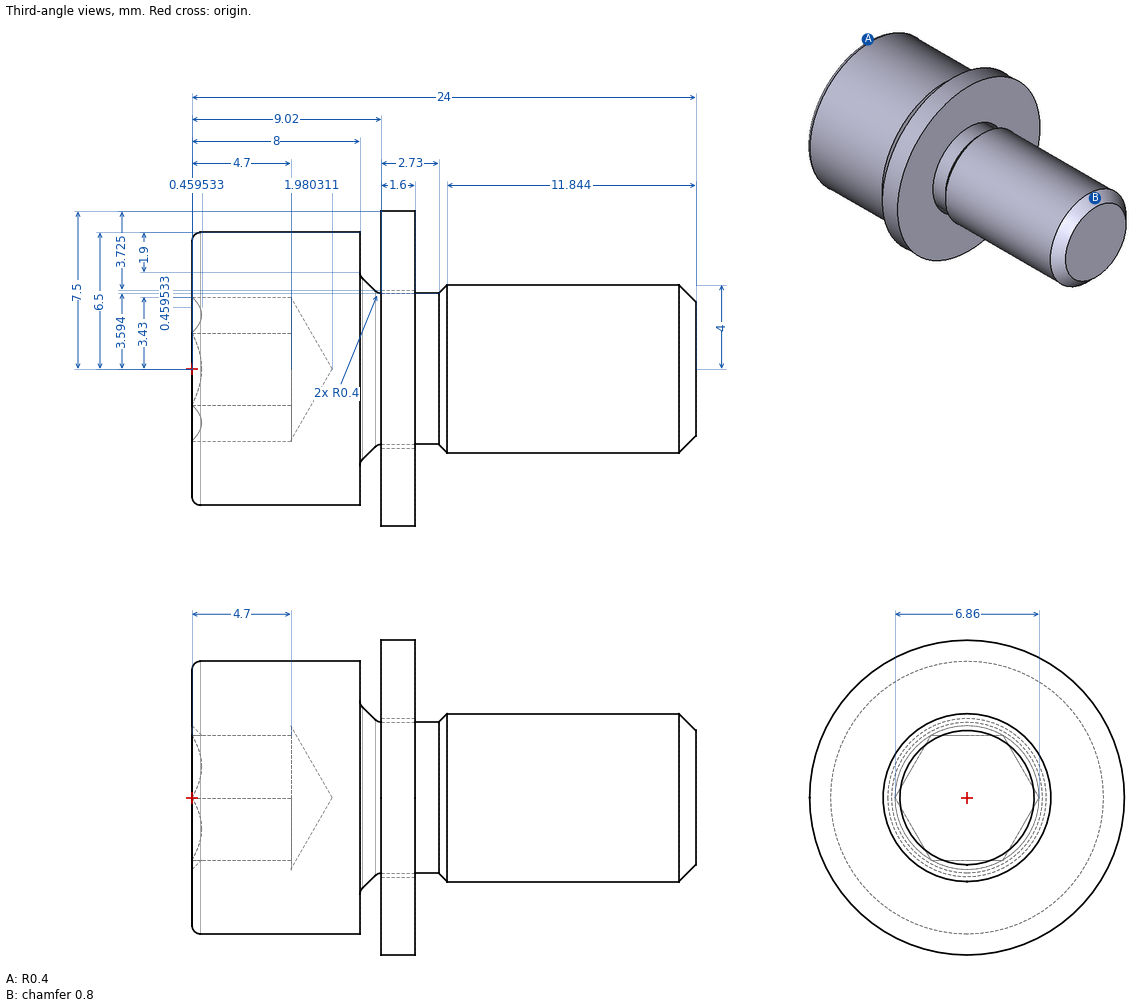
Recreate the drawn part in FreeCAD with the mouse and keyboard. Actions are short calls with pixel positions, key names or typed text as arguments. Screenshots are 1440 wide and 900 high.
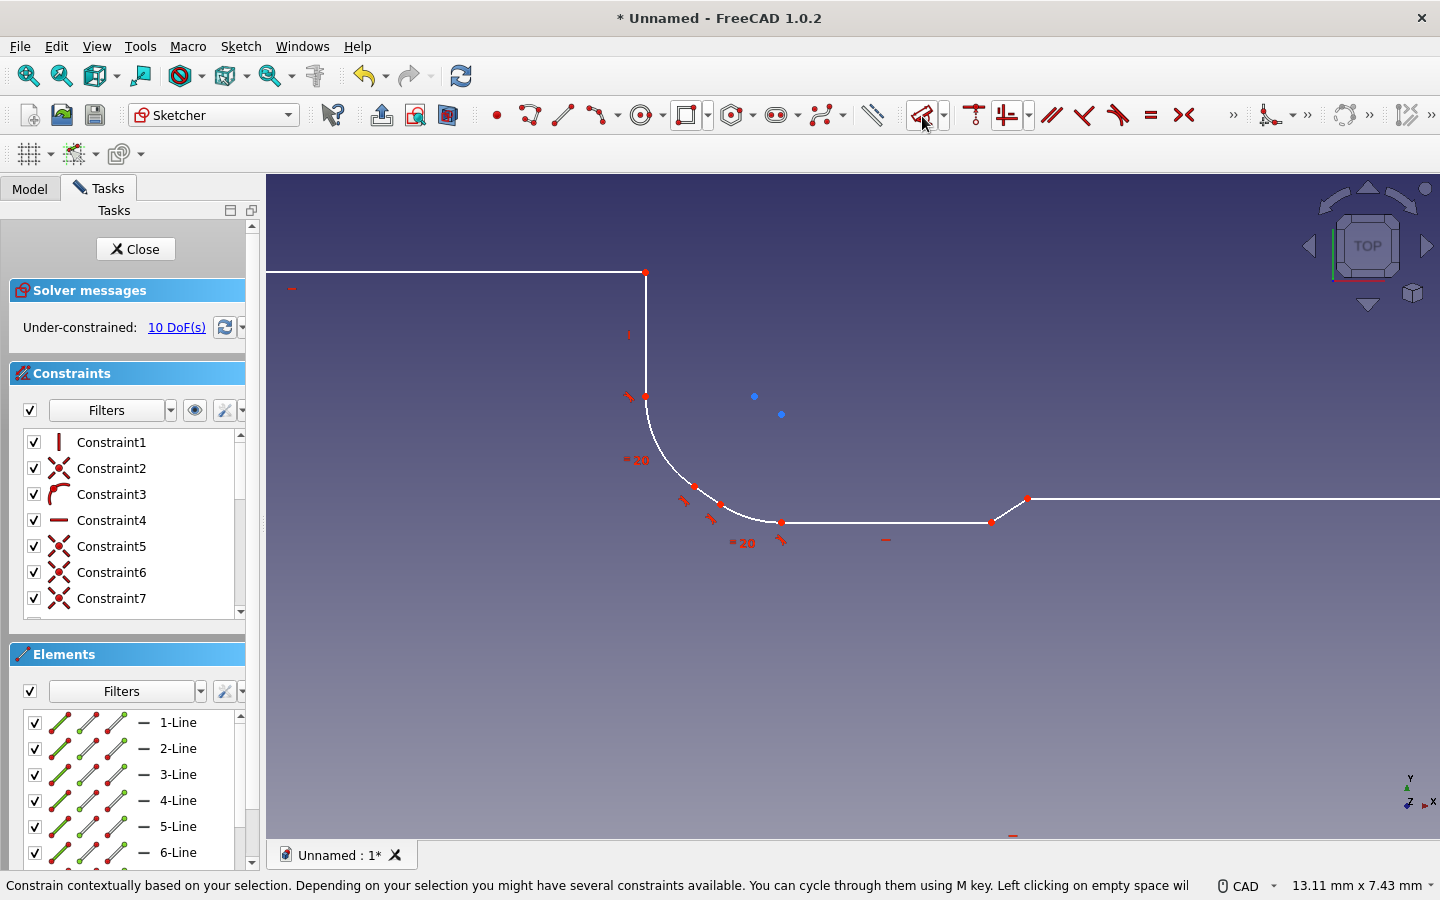
click(651, 428)
click(620, 437)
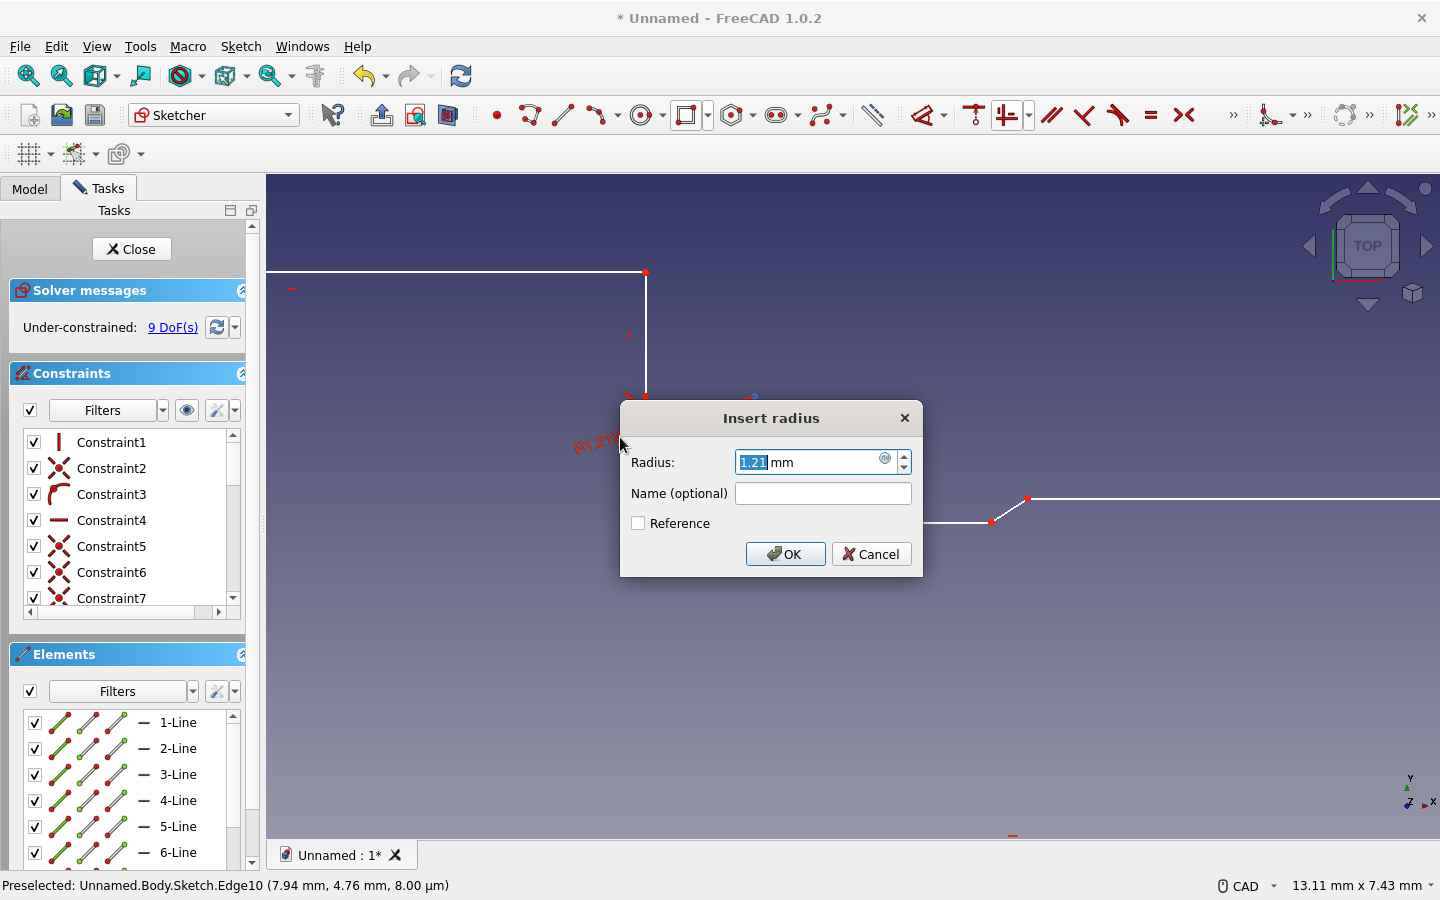
text(0.4)
key(Return)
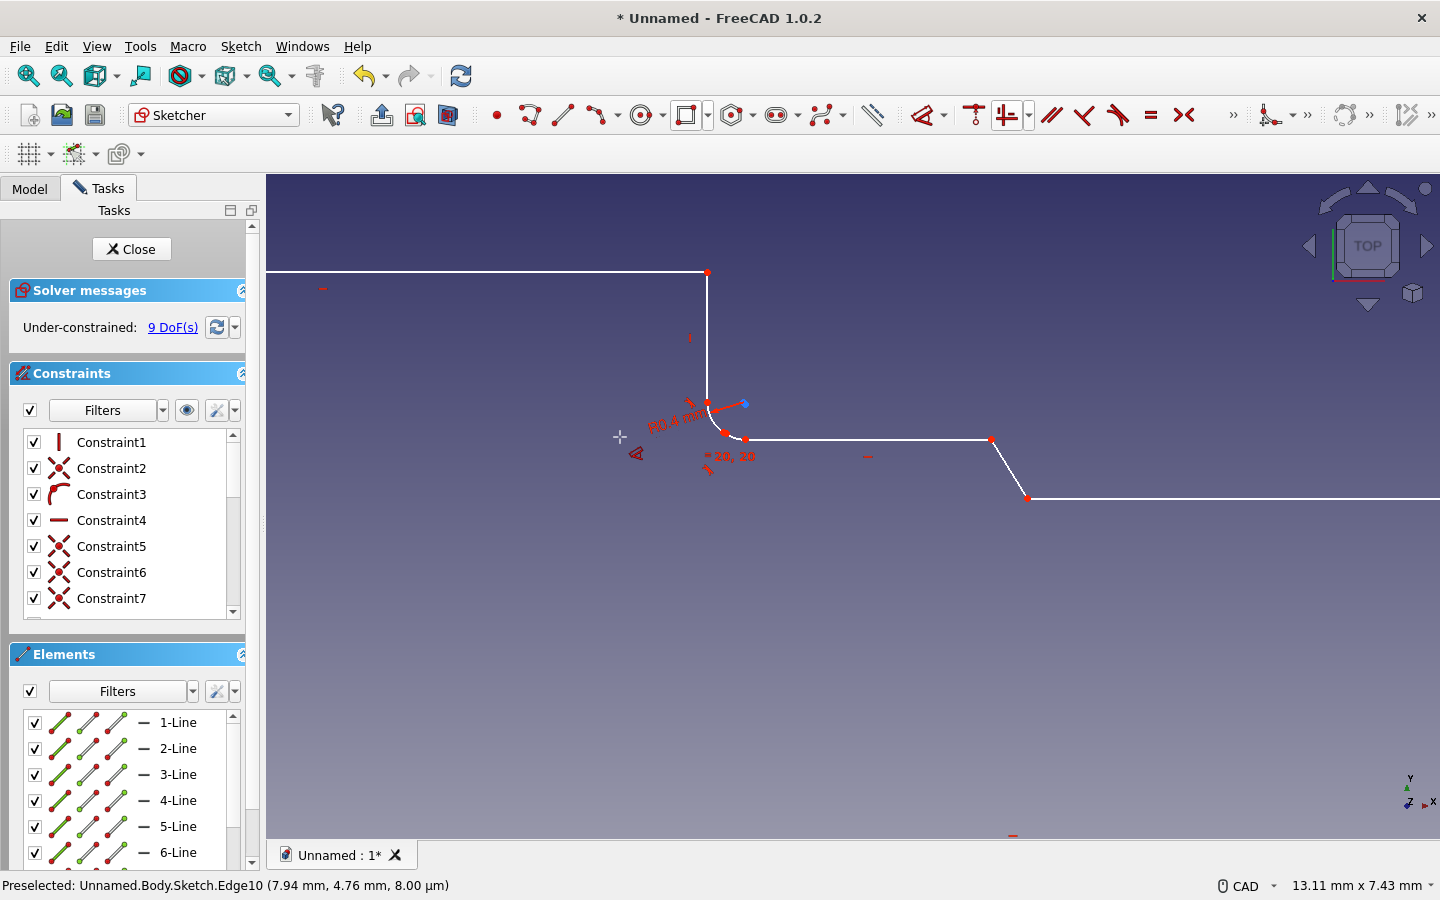
click(477, 272)
click(501, 238)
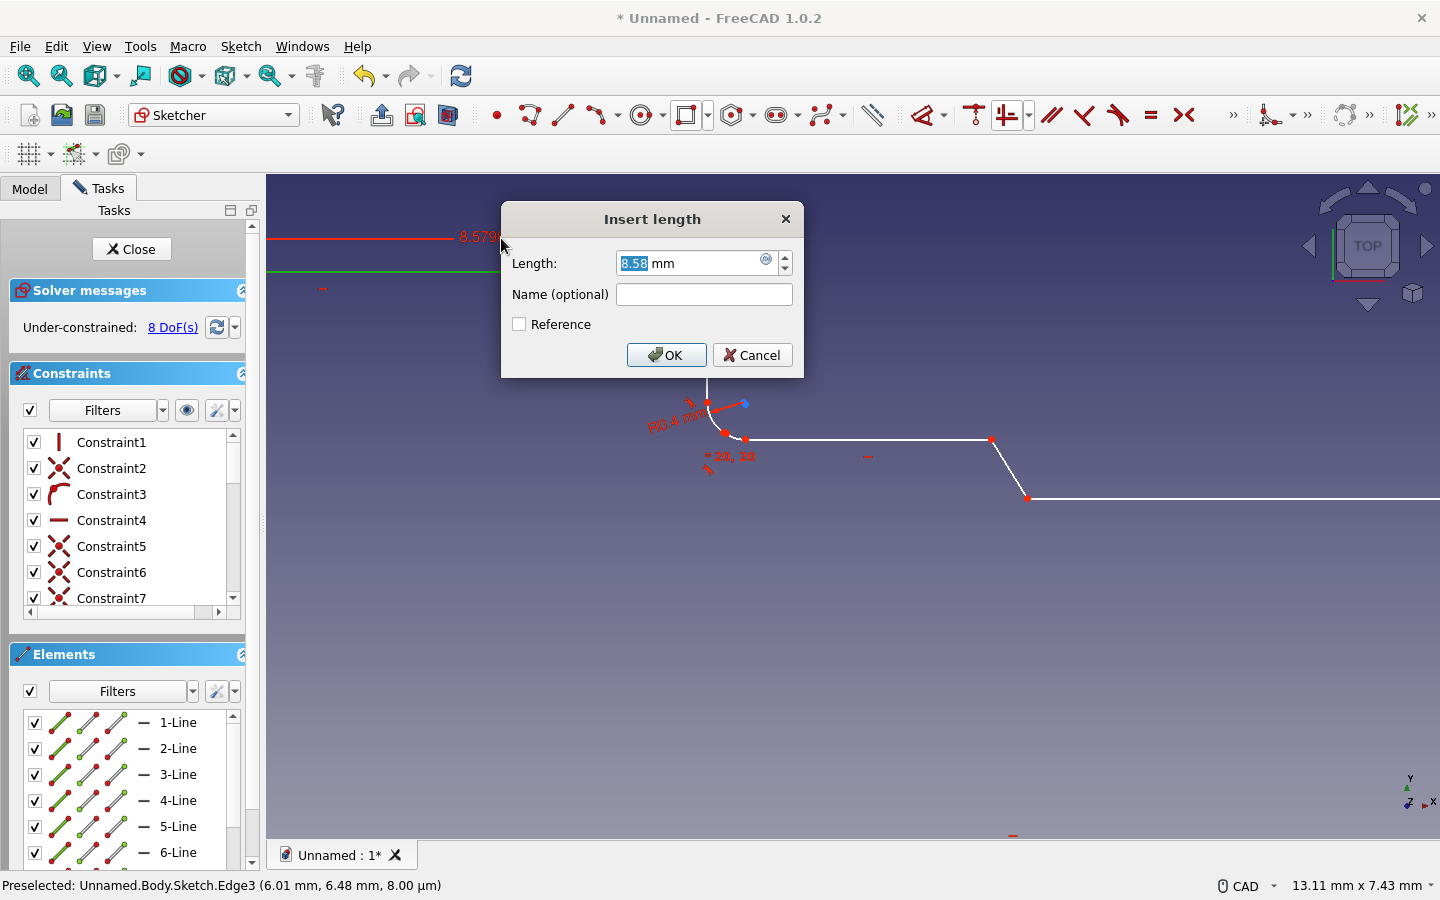
text(8)
key(Return)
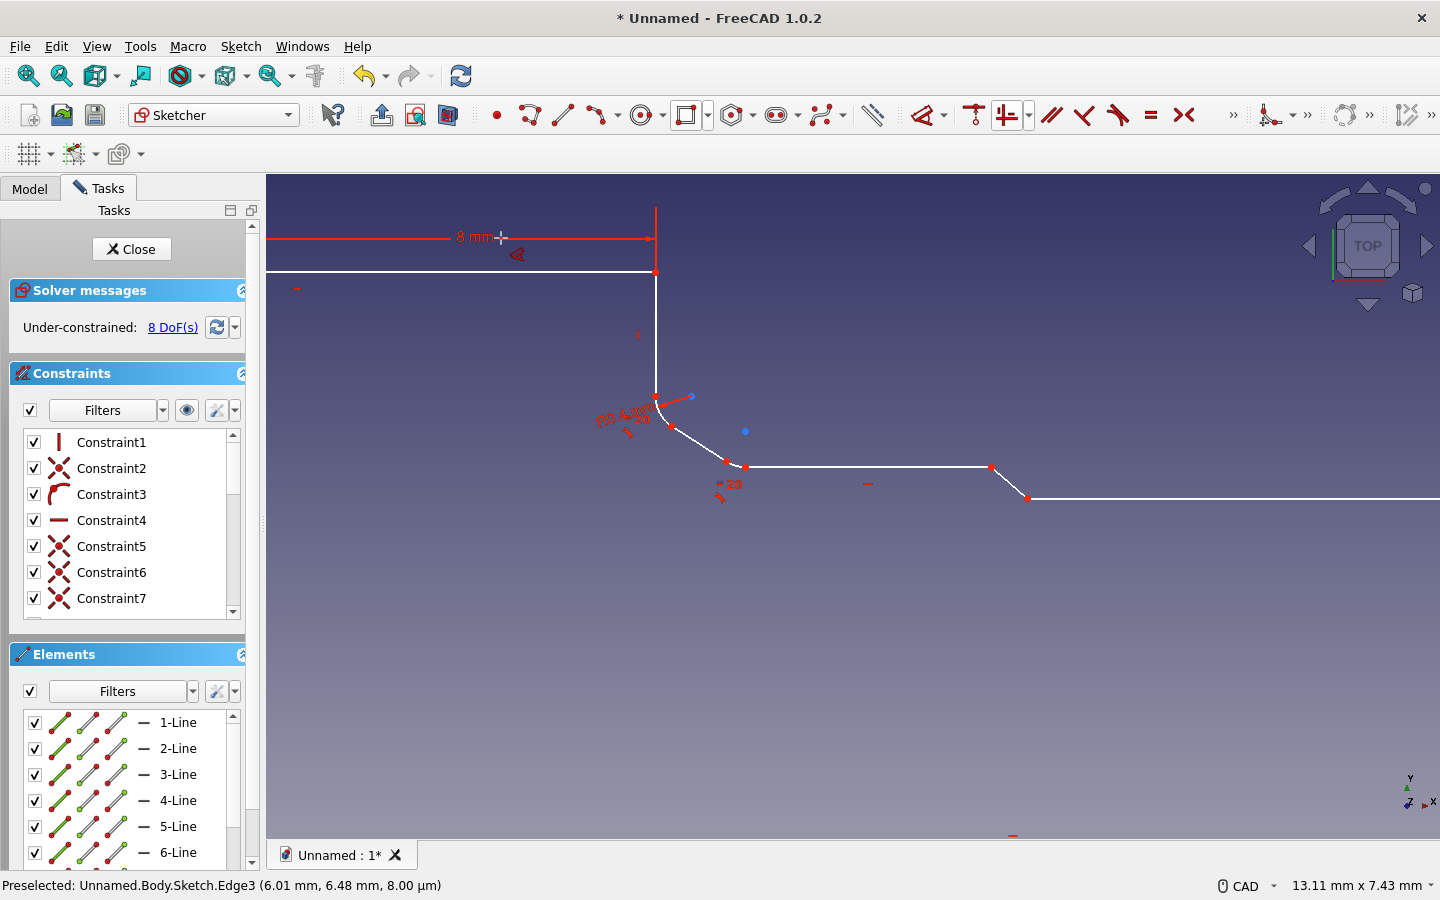
scroll(686, 483, down, 6)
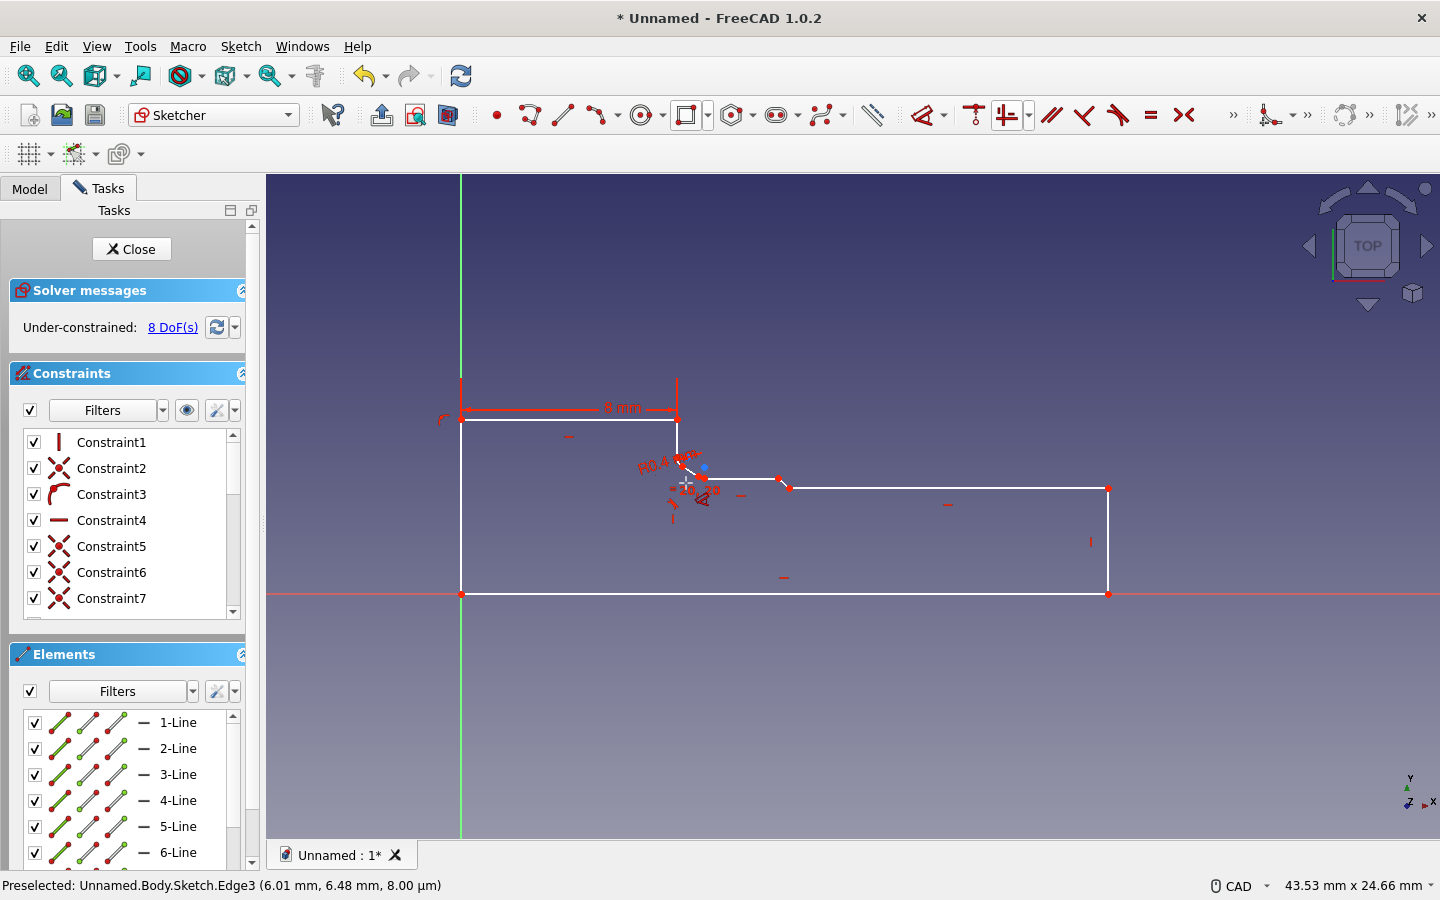
click(1108, 563)
click(1142, 541)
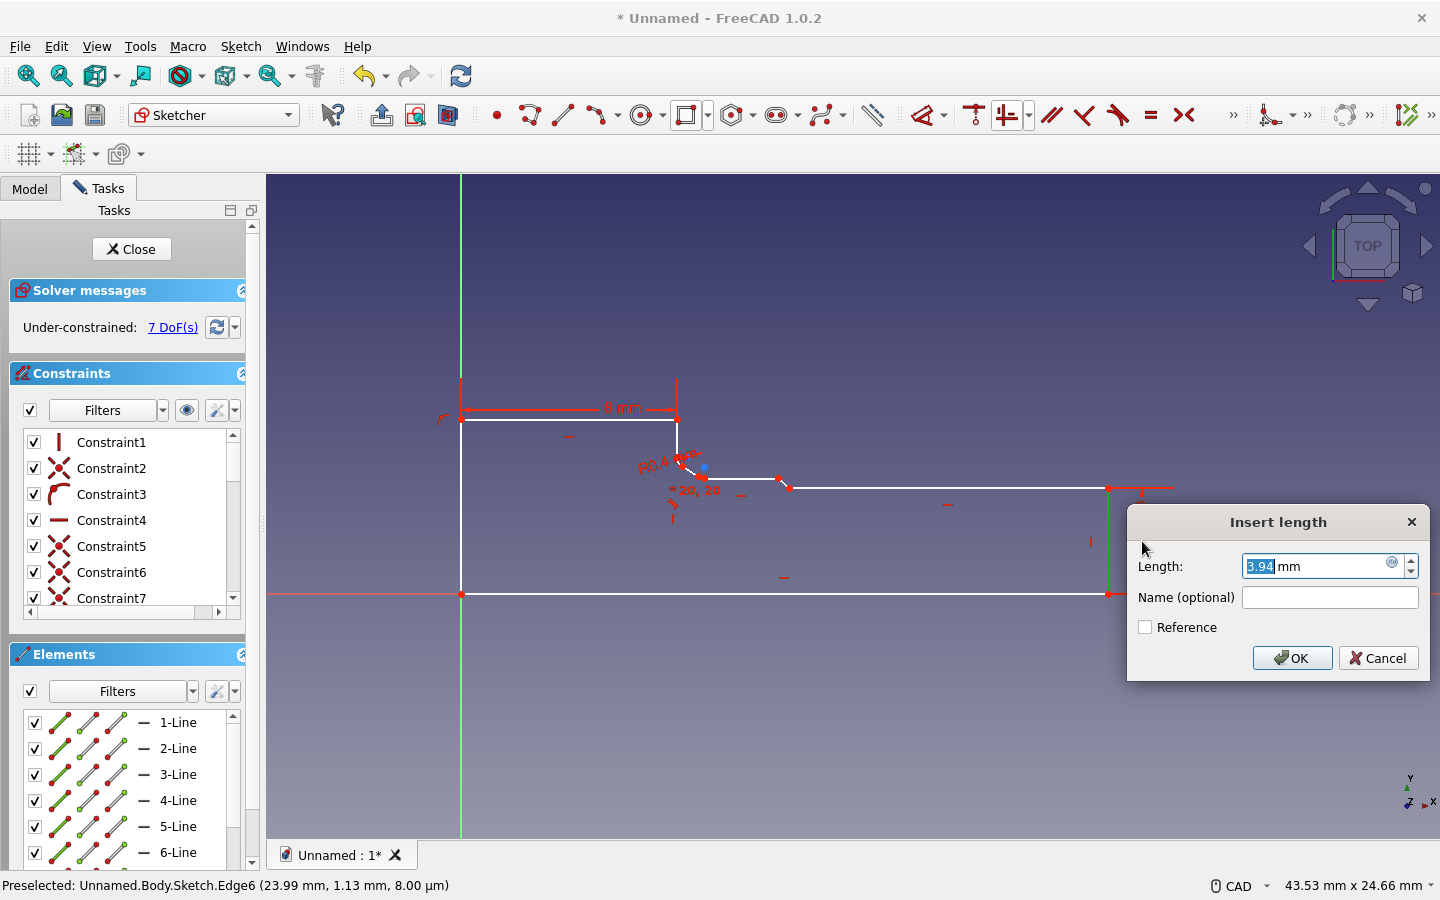
text(4)
key(Return)